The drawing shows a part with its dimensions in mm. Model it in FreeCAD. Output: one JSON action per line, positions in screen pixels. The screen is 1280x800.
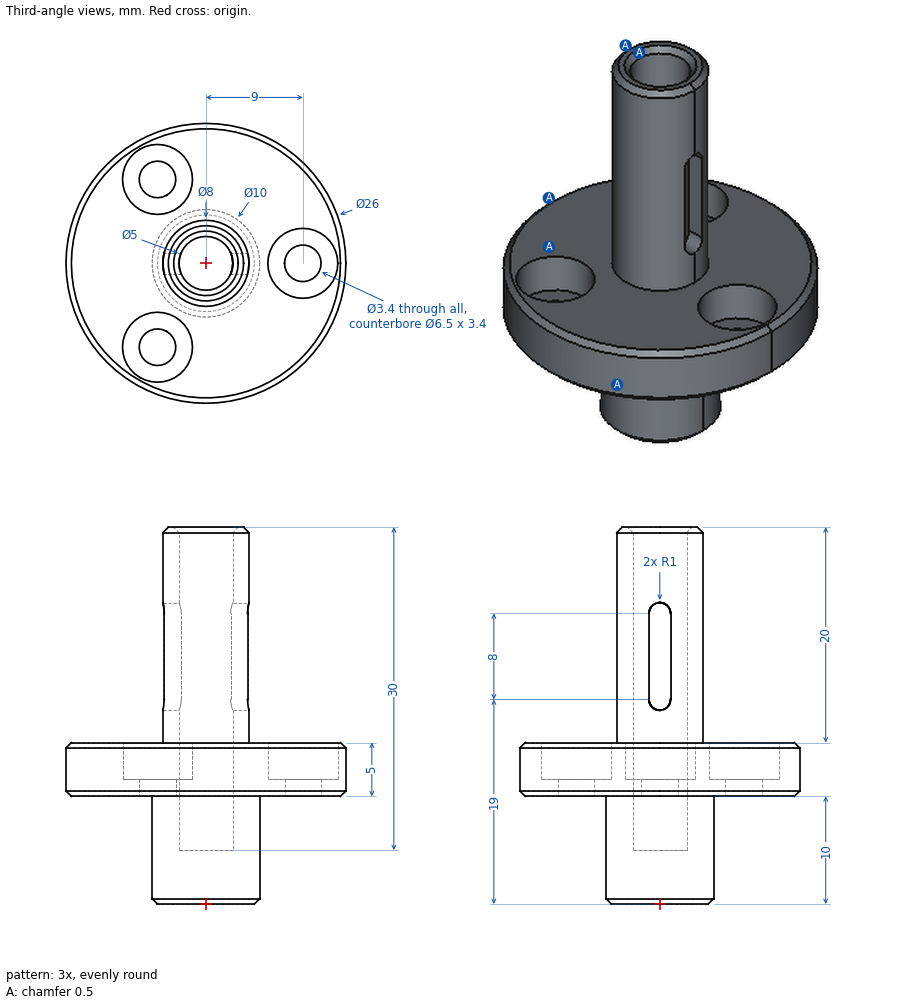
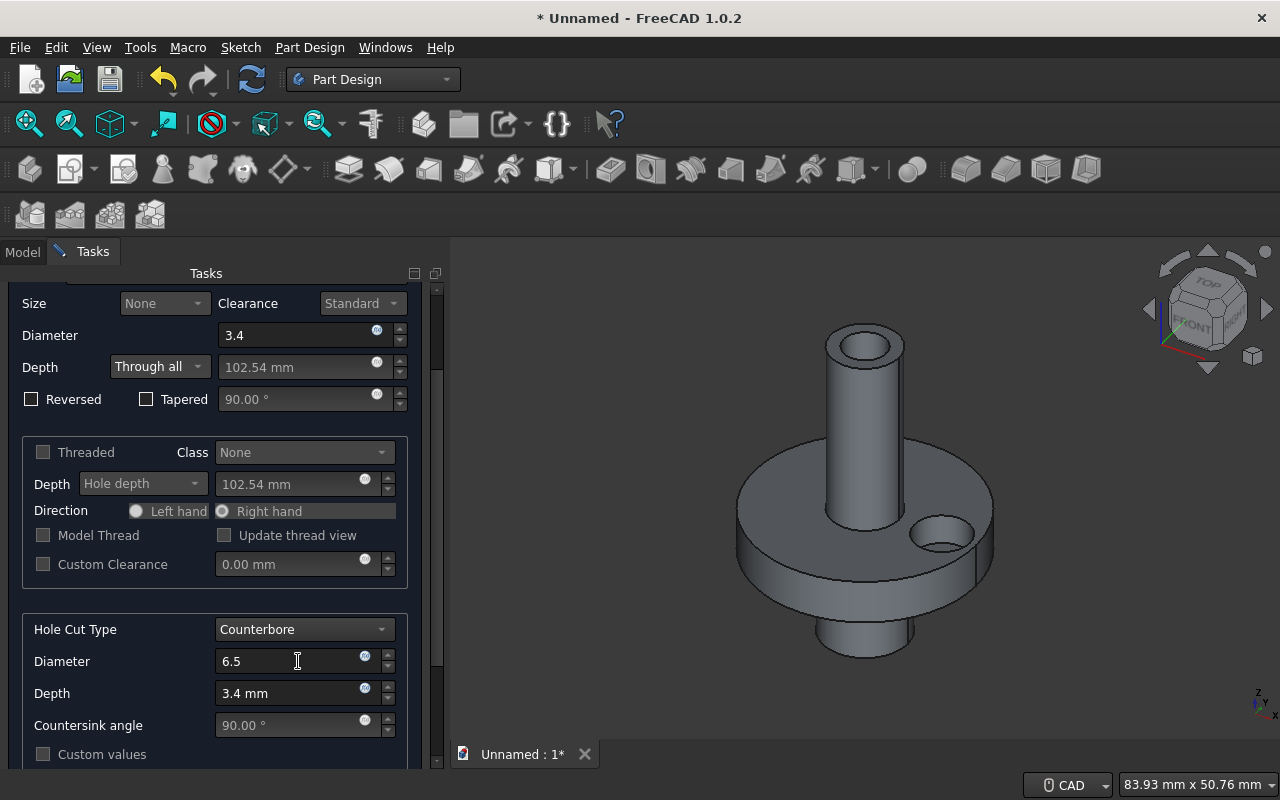
{"action": "scroll", "coordinate": [437, 526], "scroll_direction": "up", "scroll_amount": 3}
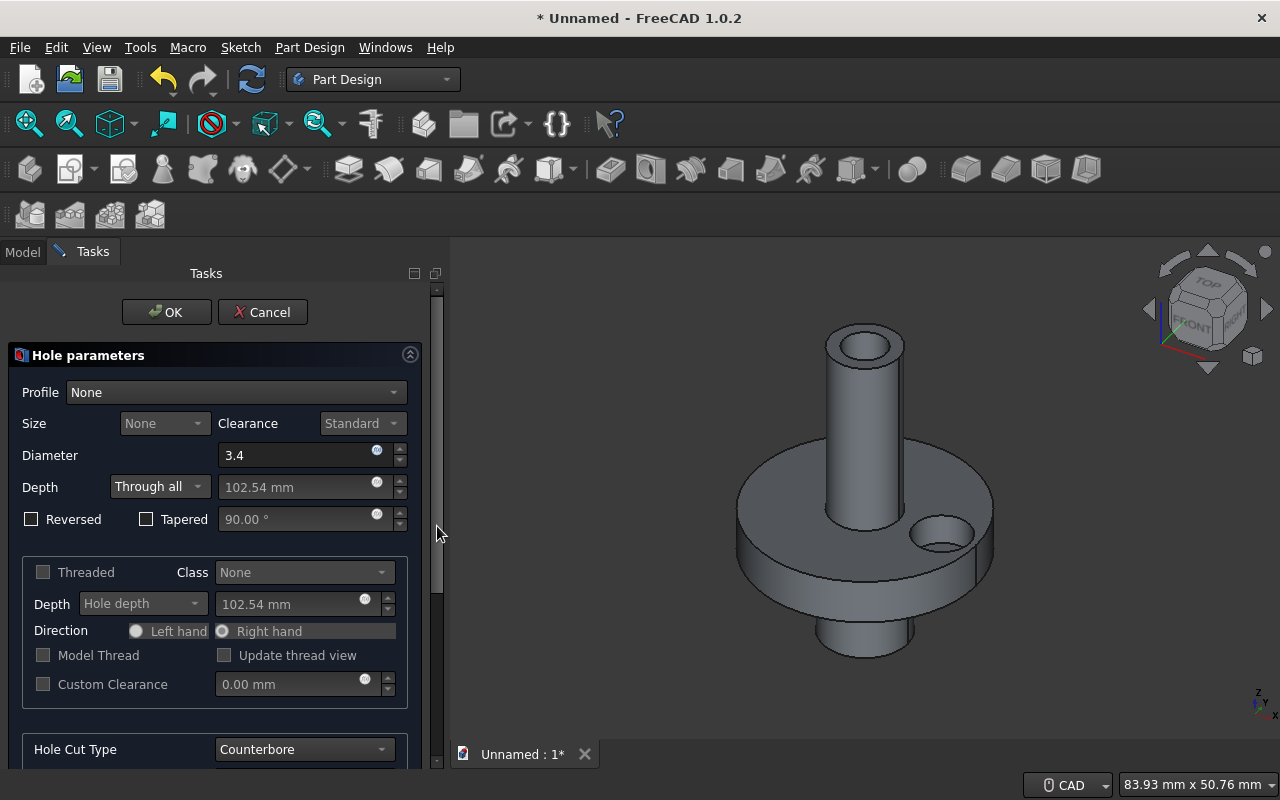
{"action": "left_click", "coordinate": [167, 312]}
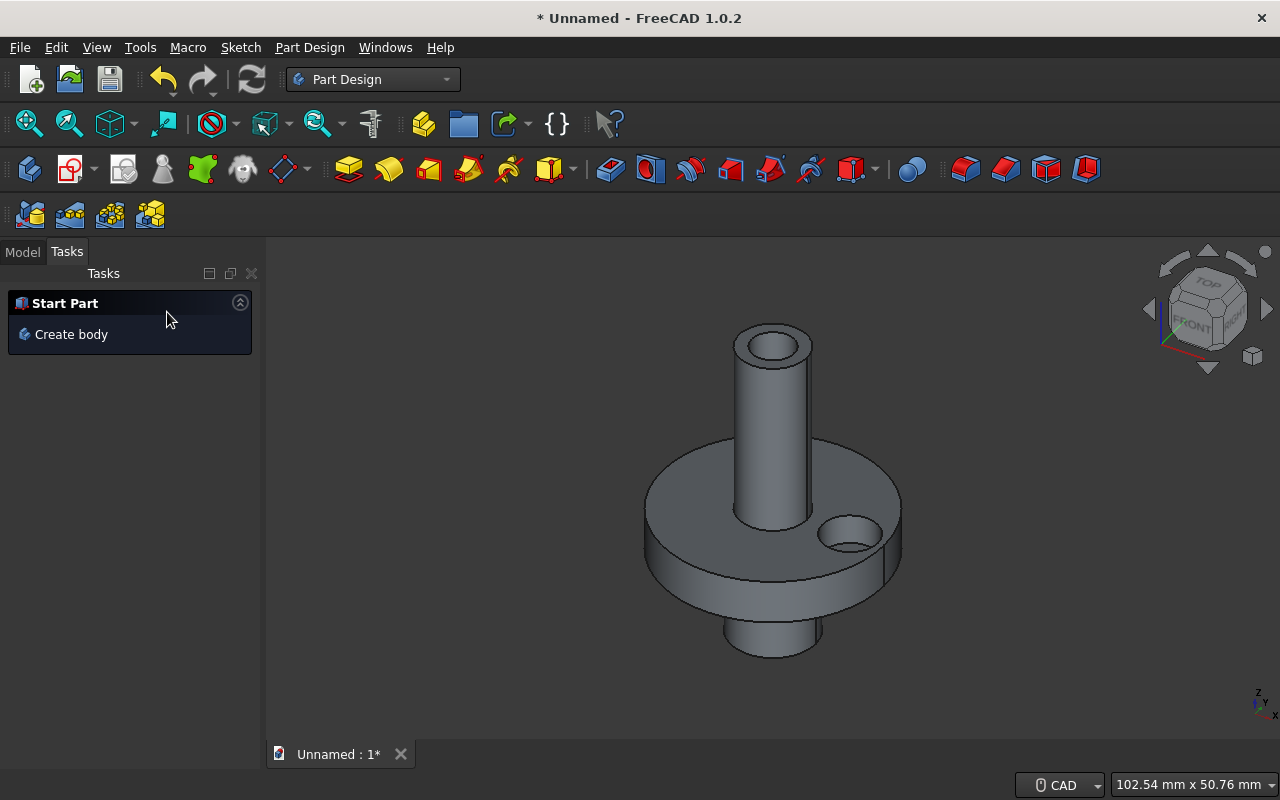
{"action": "left_click", "coordinate": [23, 251]}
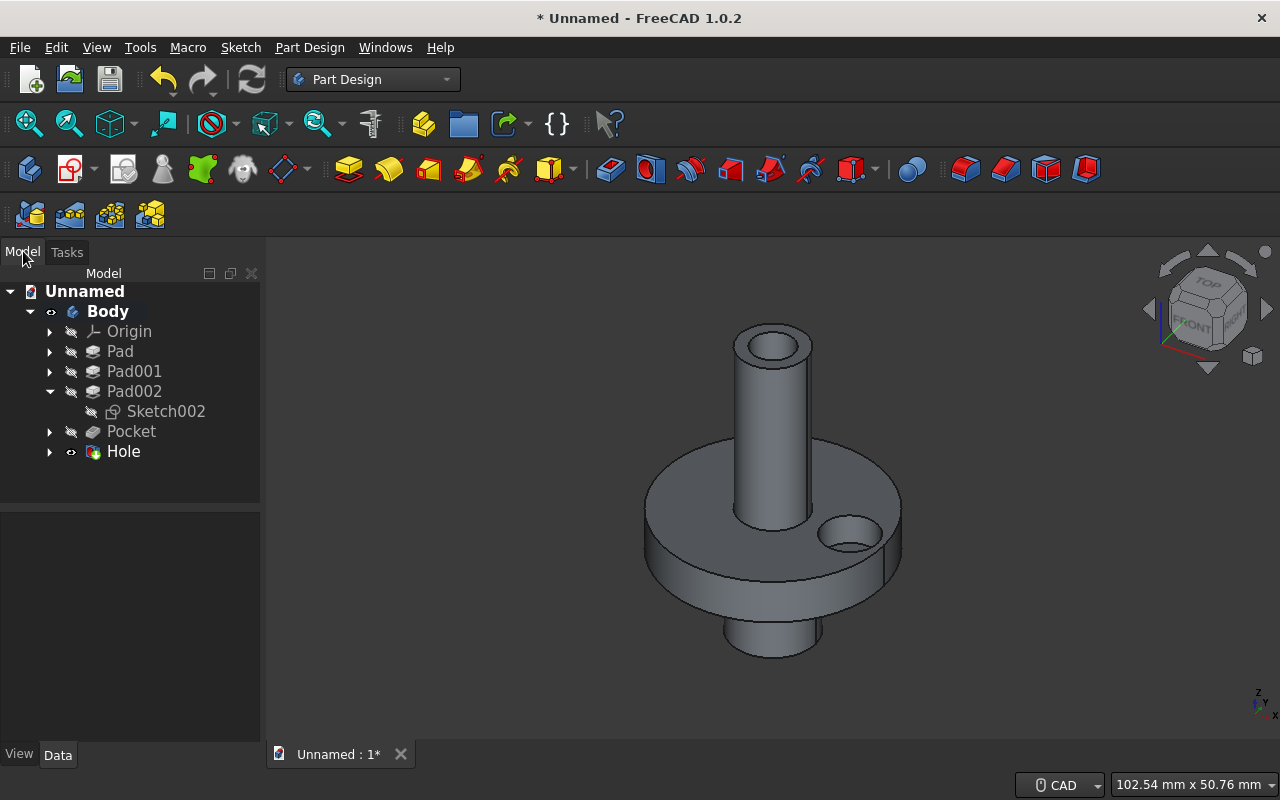
{"action": "left_click", "coordinate": [116, 452]}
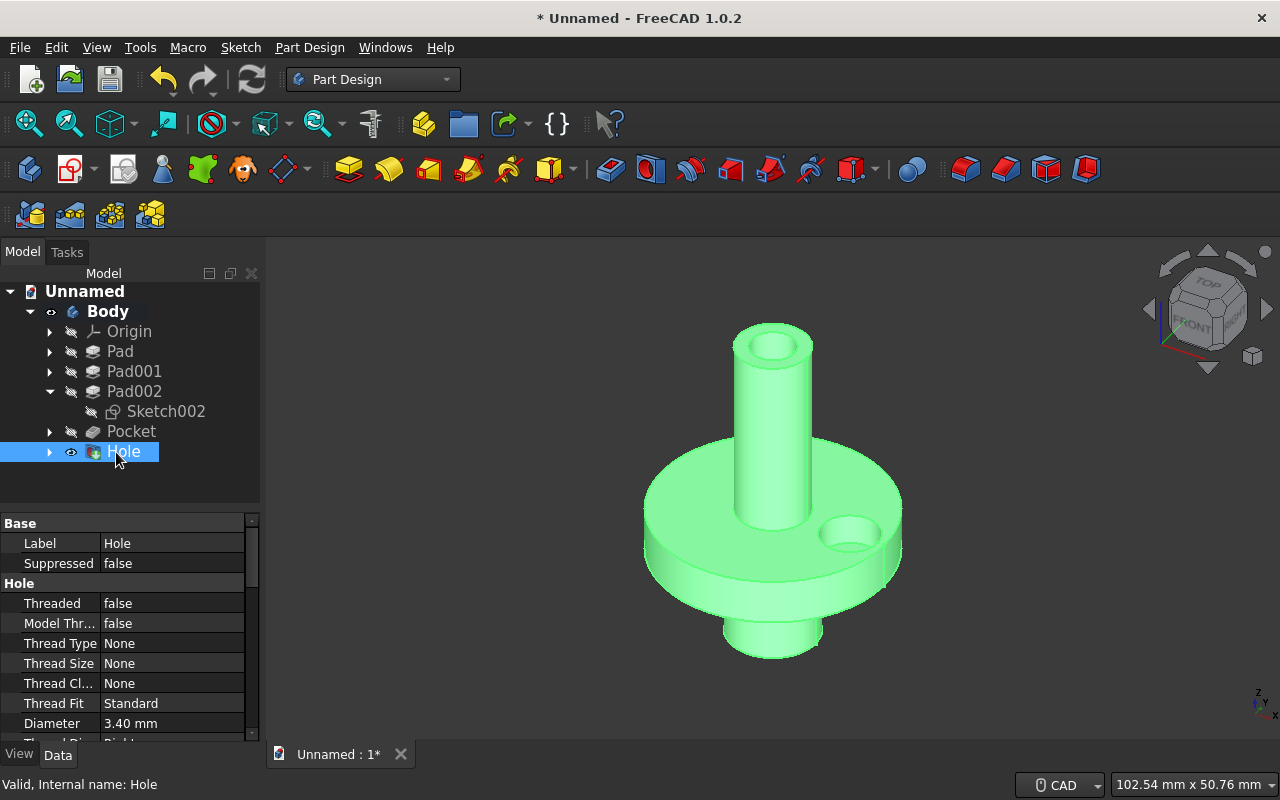
{"action": "left_click", "coordinate": [110, 214]}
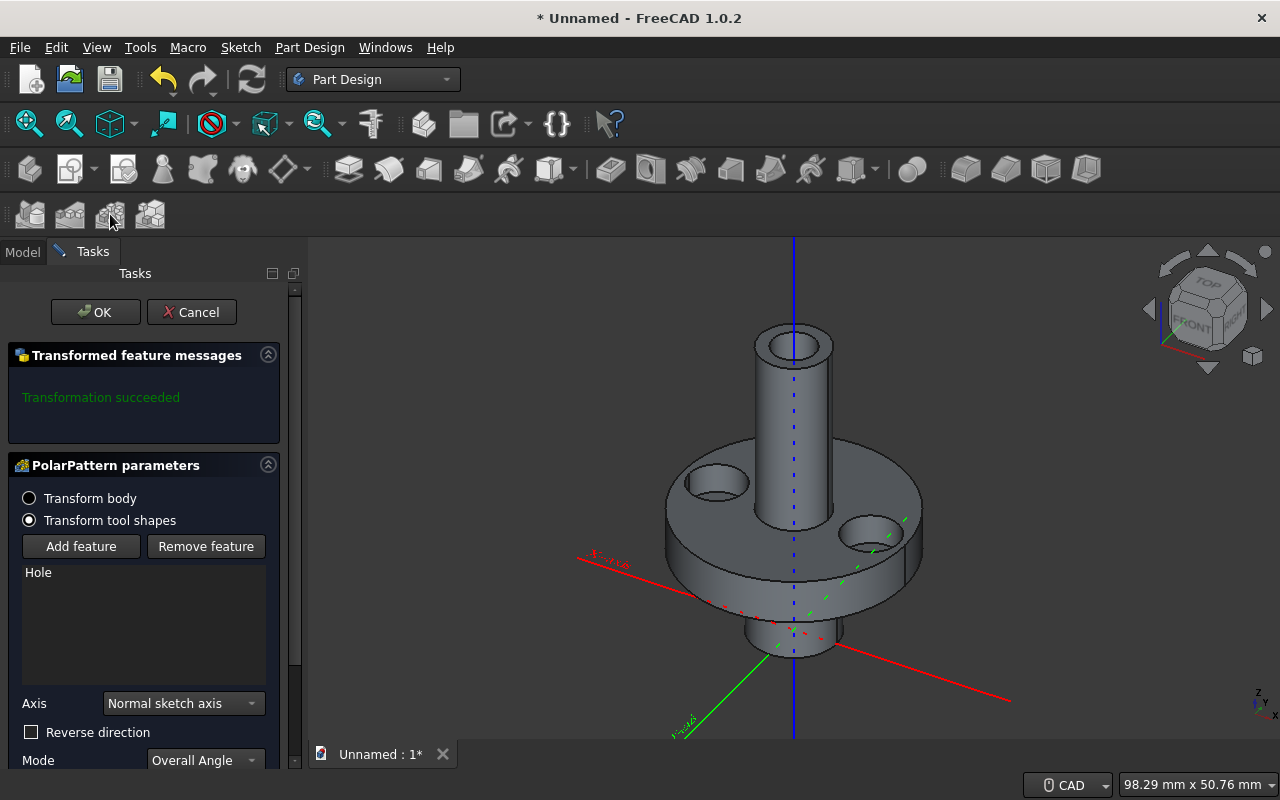
{"action": "left_click", "coordinate": [184, 704]}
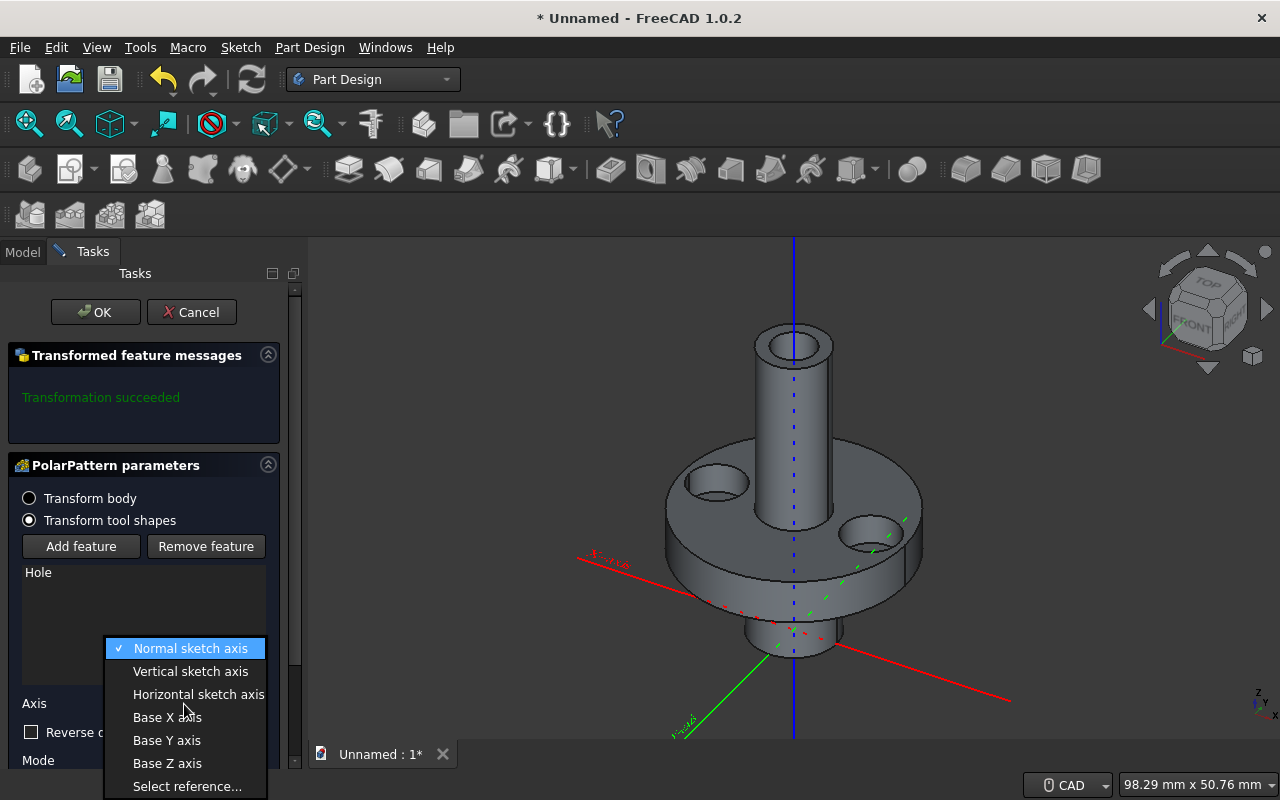
{"action": "left_click", "coordinate": [184, 764]}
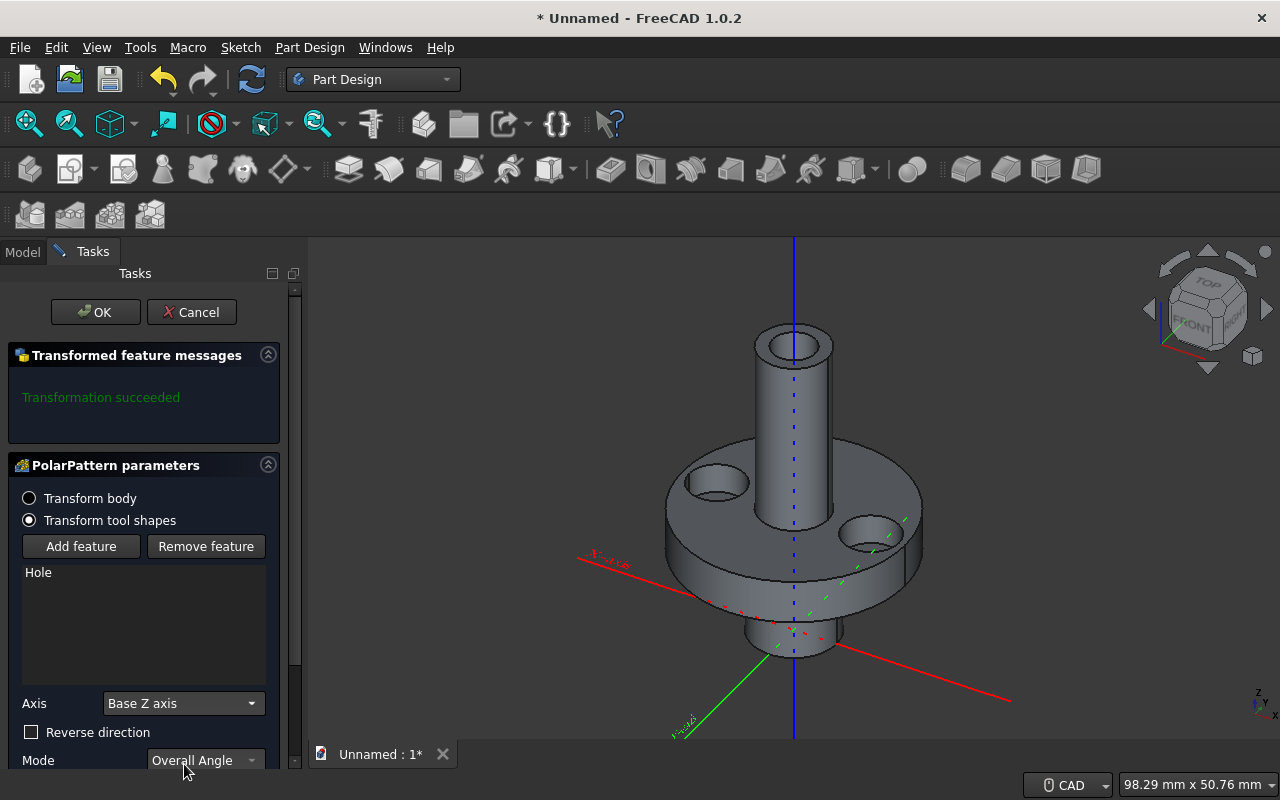
{"action": "scroll", "coordinate": [295, 526], "scroll_direction": "down", "scroll_amount": 3}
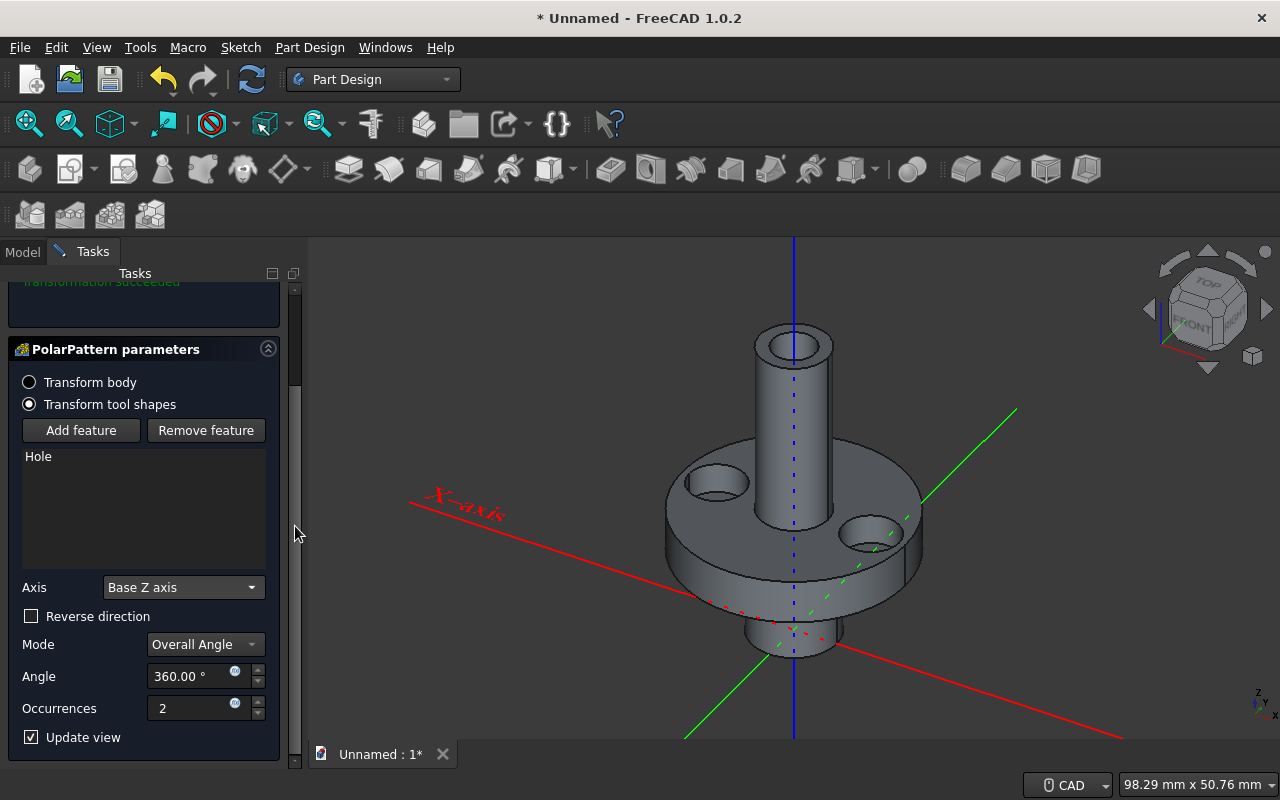
{"action": "triple_click", "coordinate": [198, 708]}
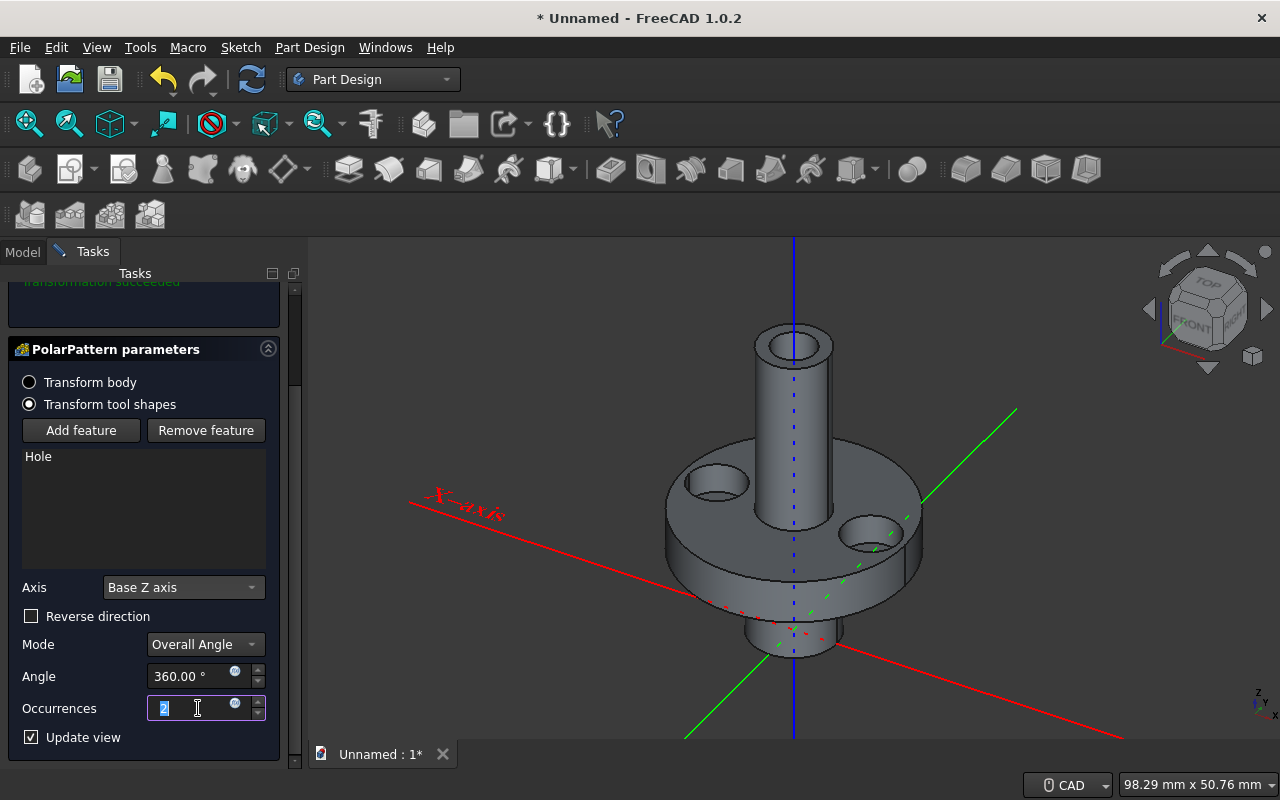
{"action": "type", "text": "3"}
{"action": "key", "text": "Tab"}